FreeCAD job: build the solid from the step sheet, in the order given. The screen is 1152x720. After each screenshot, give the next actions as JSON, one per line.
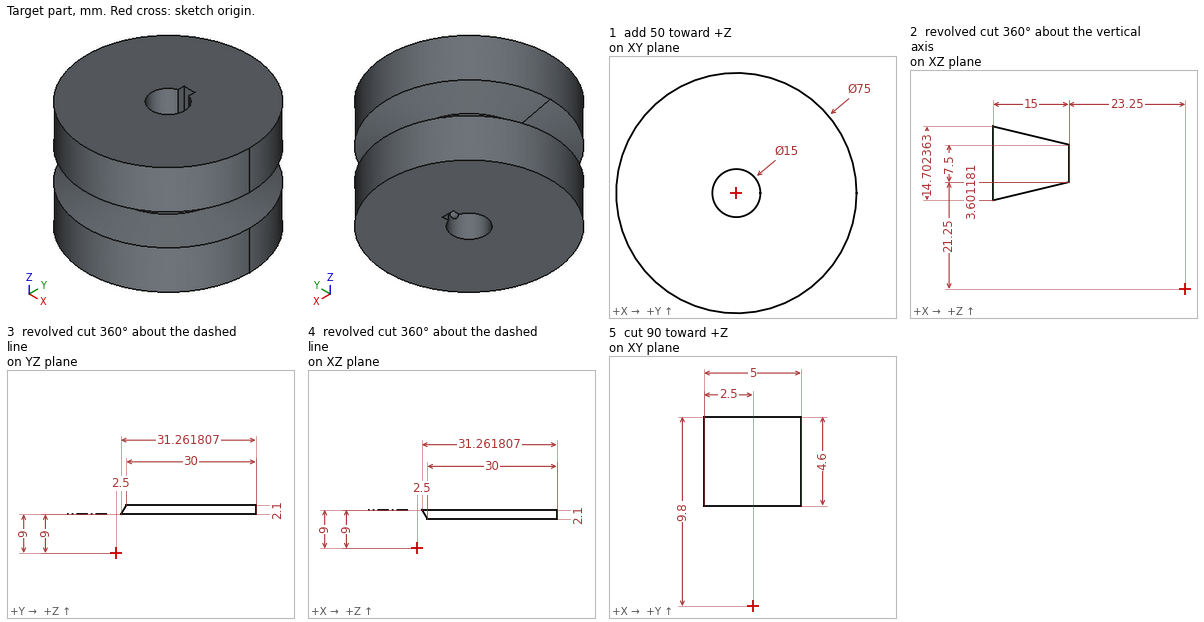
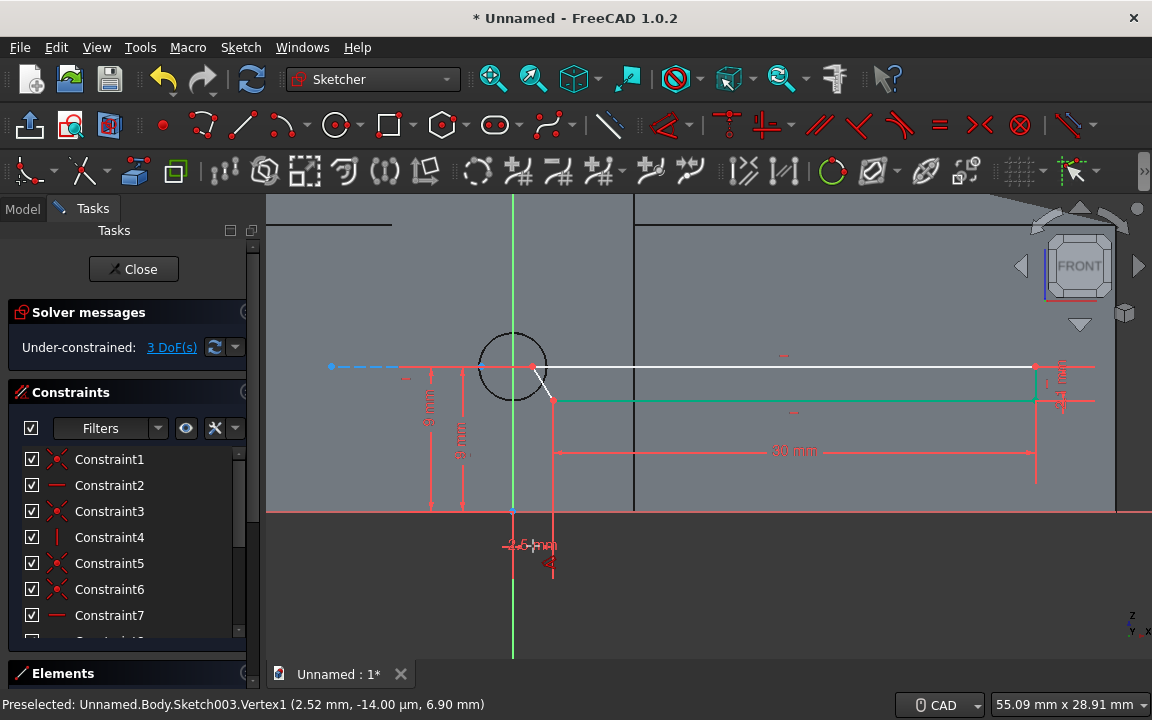
{"action": "left_click", "coordinate": [684, 367]}
{"action": "left_click", "coordinate": [760, 333]}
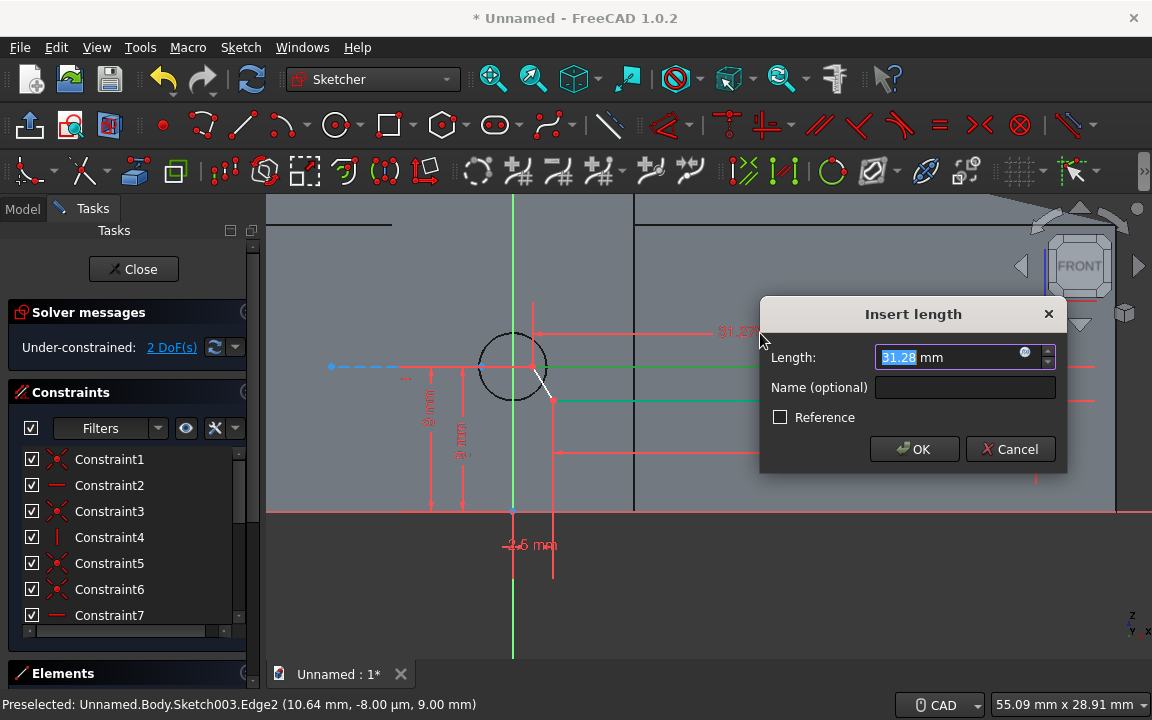
{"action": "type", "text": "31.261807"}
{"action": "key", "text": "Return"}
{"action": "key", "text": "Escape"}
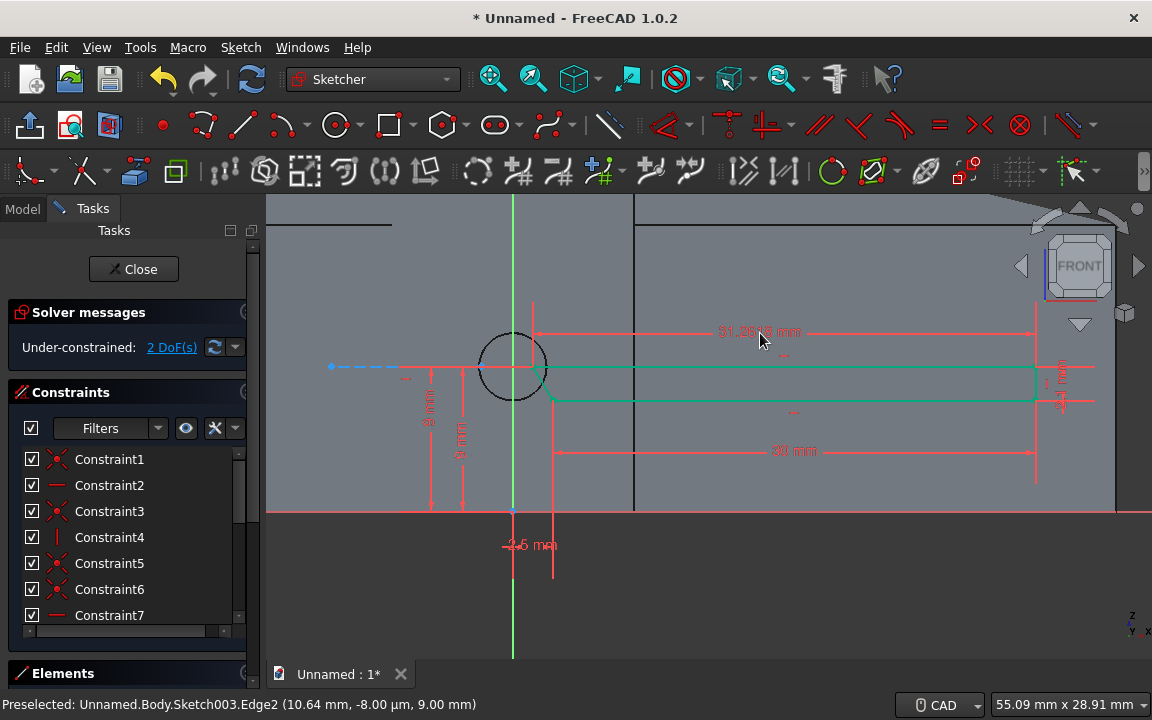
{"action": "left_click", "coordinate": [134, 269]}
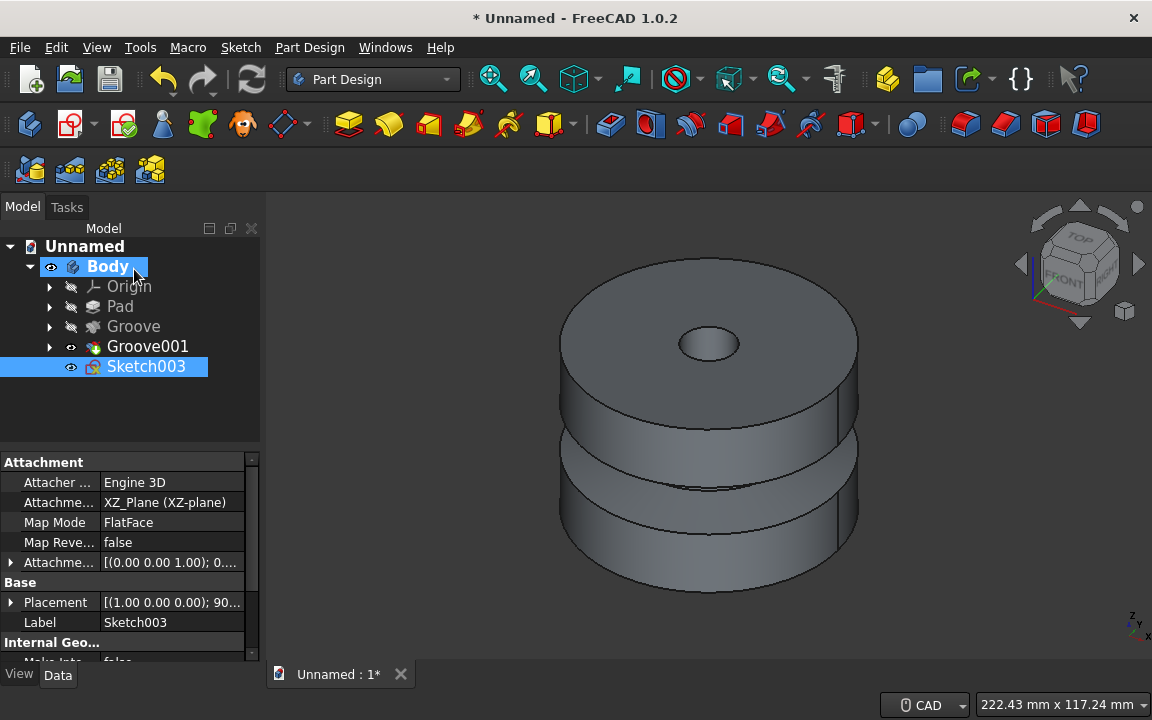
{"action": "left_click", "coordinate": [692, 124]}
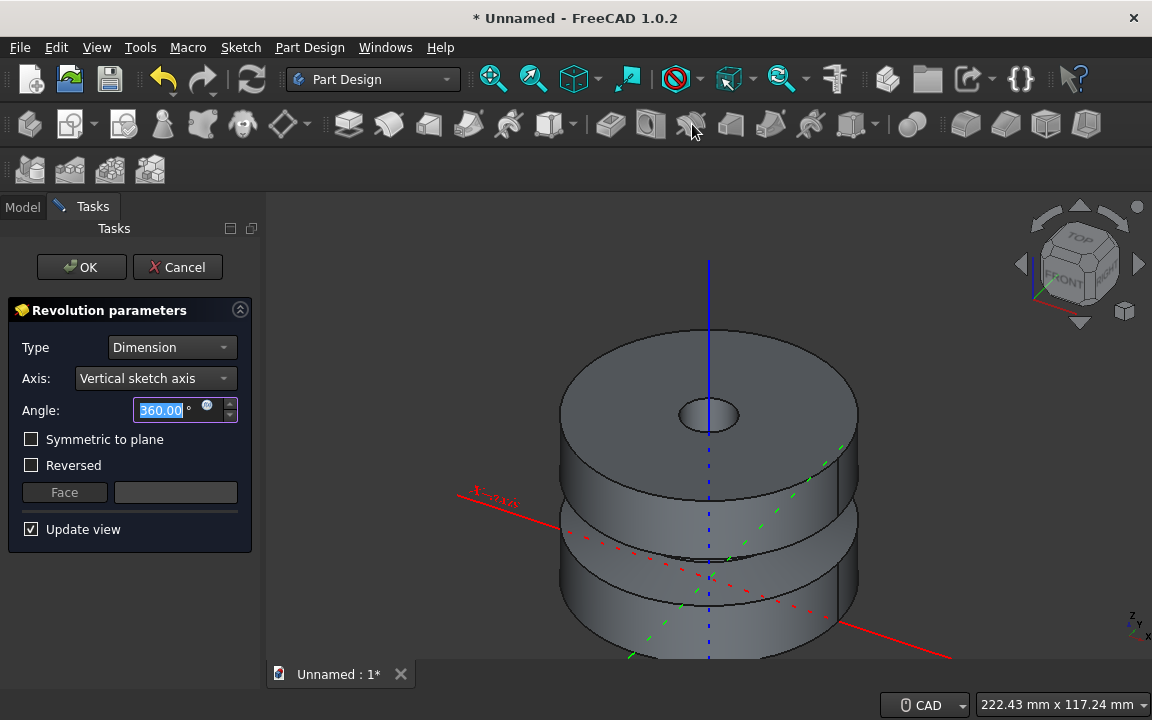
{"action": "left_click", "coordinate": [156, 378]}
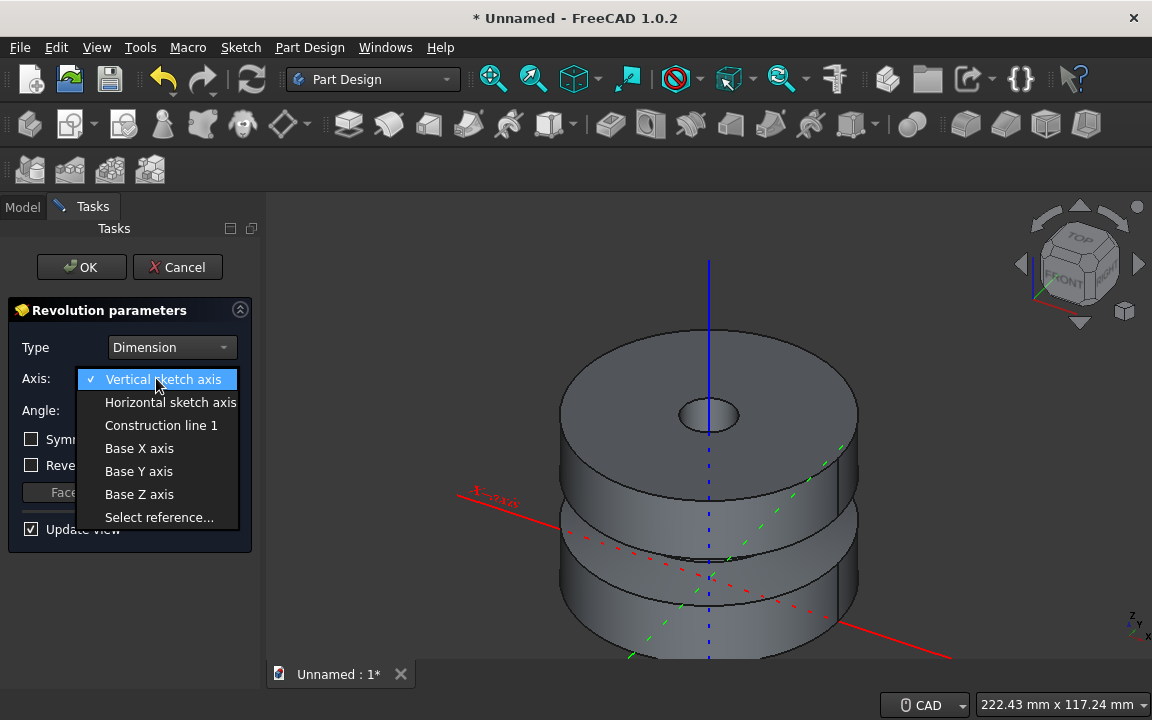
{"action": "left_click", "coordinate": [156, 426]}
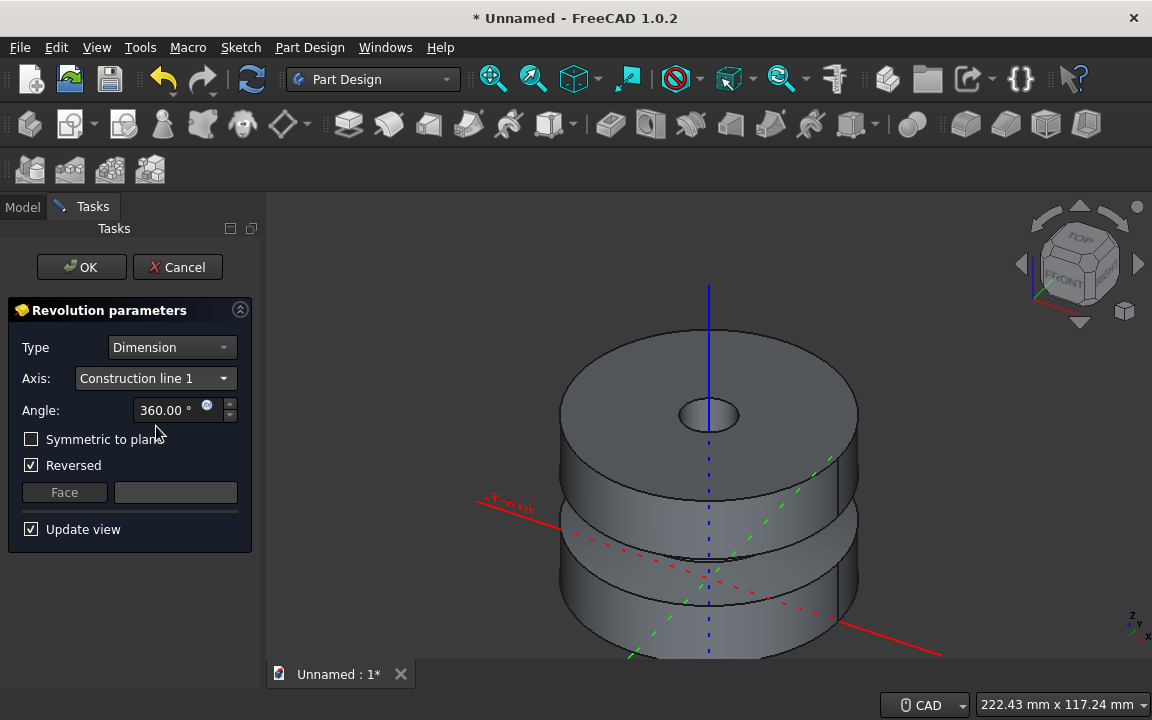
{"action": "left_click", "coordinate": [82, 267]}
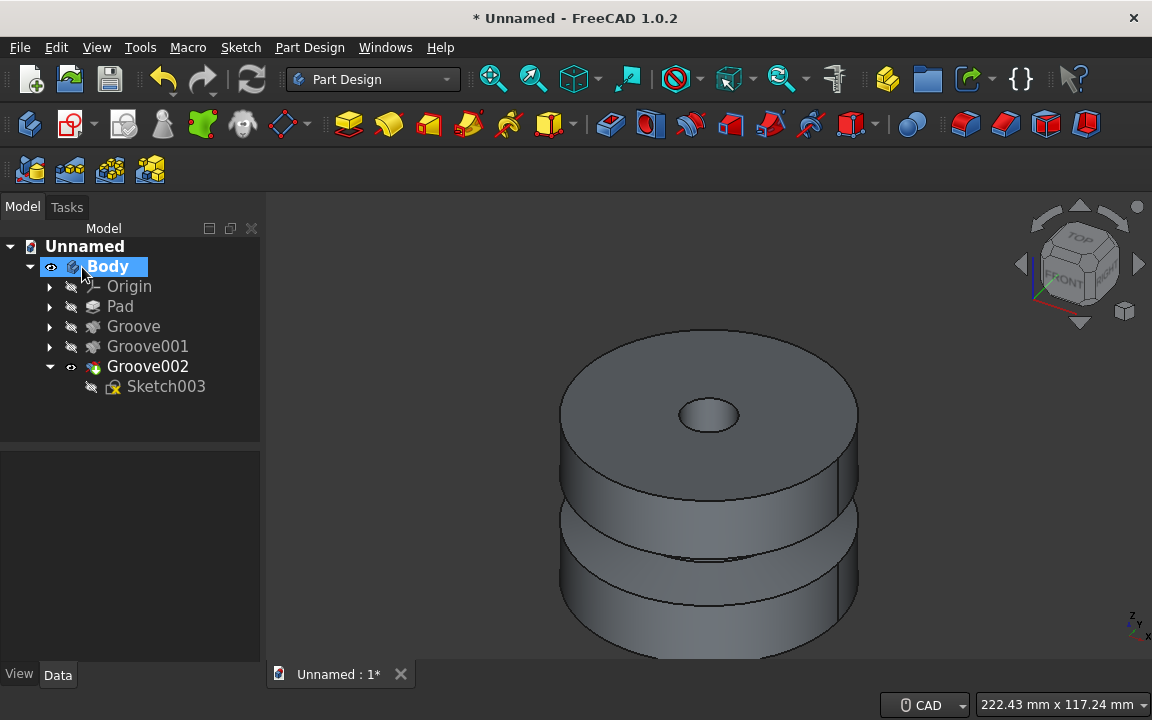
{"action": "left_click", "coordinate": [494, 80]}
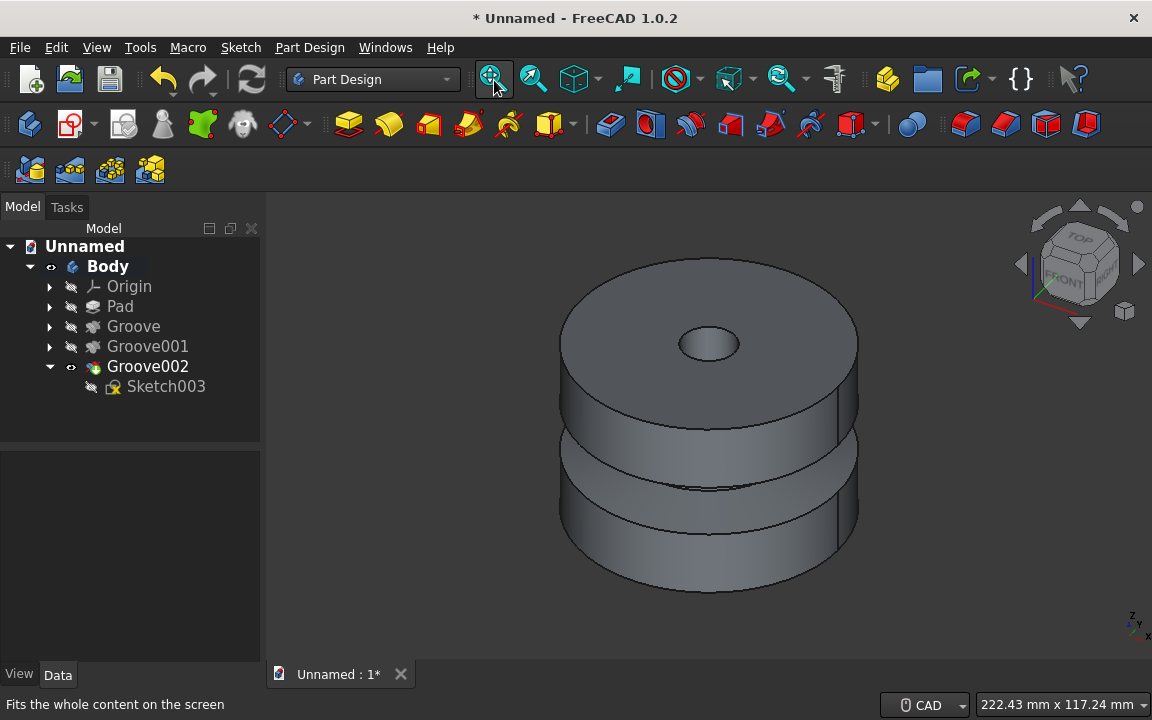
{"action": "left_click", "coordinate": [70, 124]}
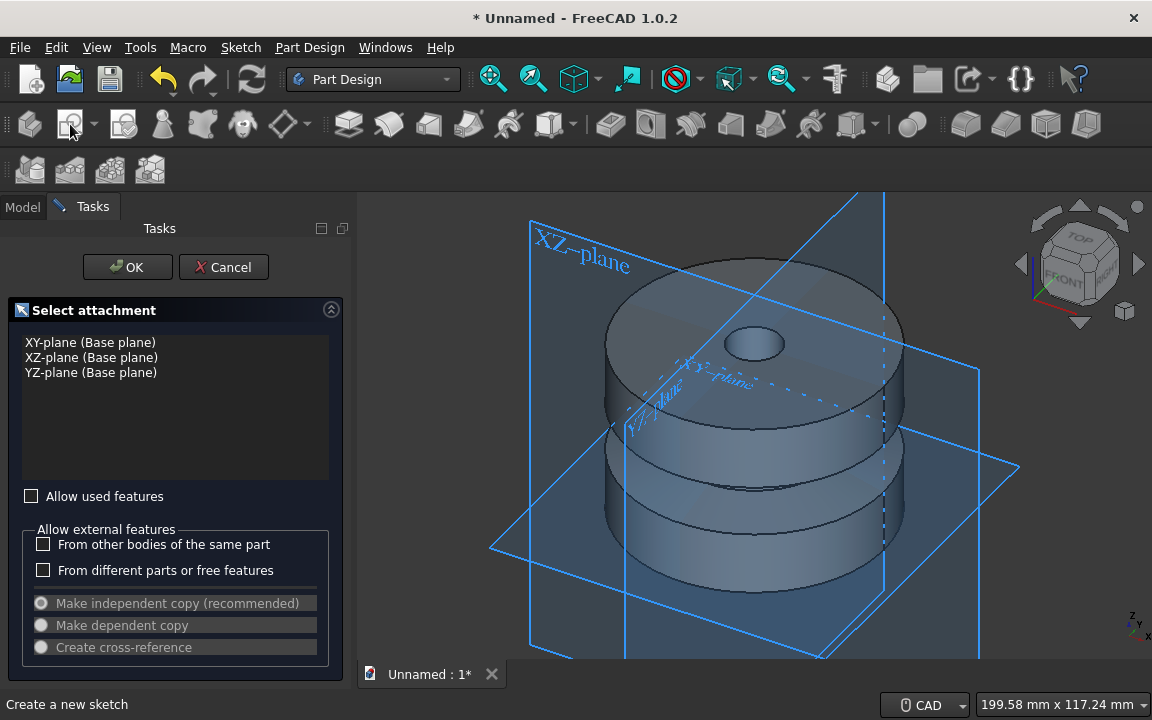
{"action": "left_click", "coordinate": [82, 342]}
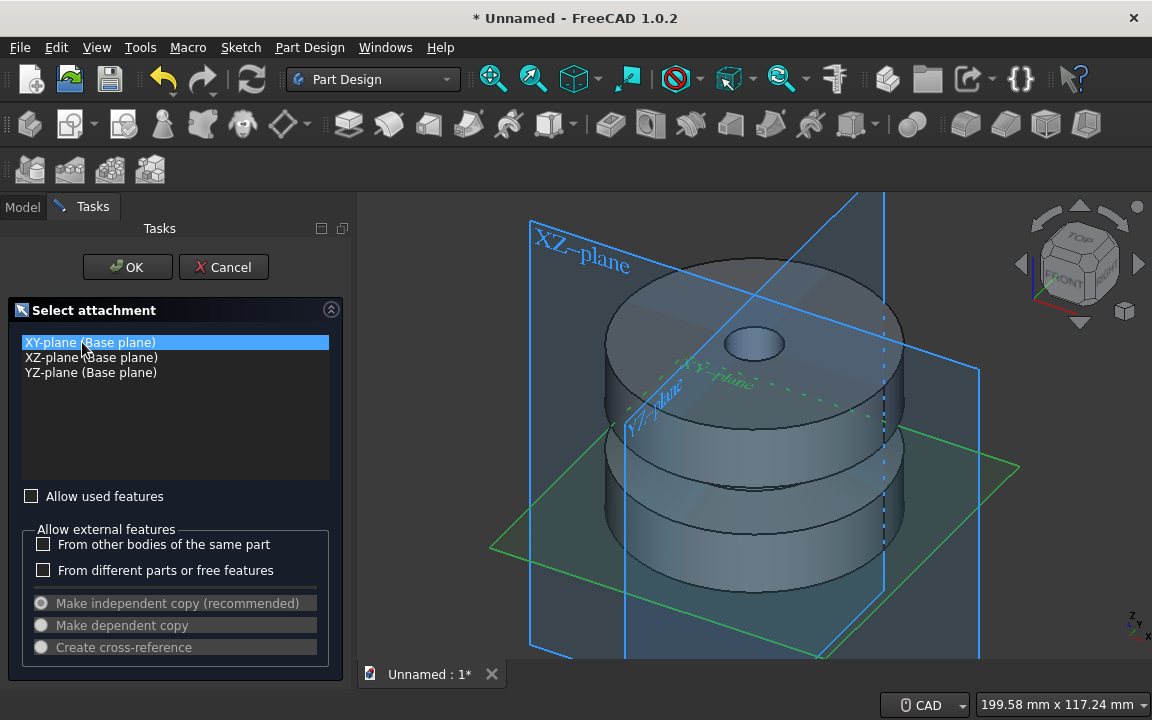
{"action": "left_click", "coordinate": [128, 267]}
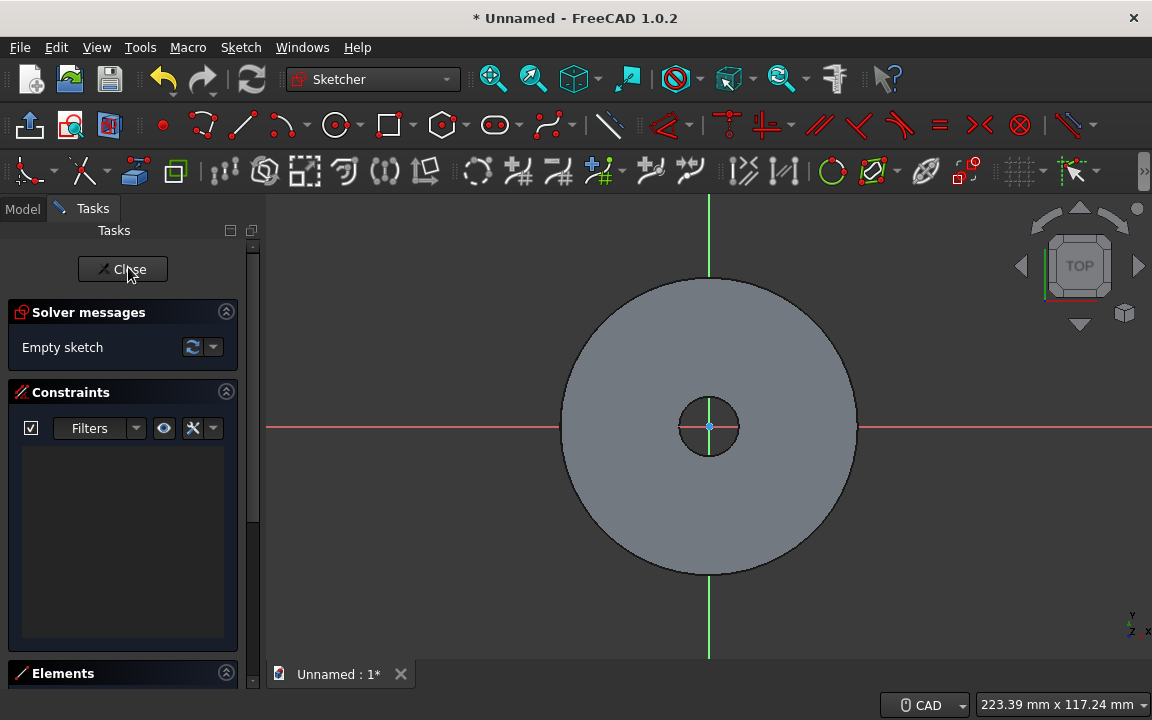
{"action": "left_click", "coordinate": [110, 126]}